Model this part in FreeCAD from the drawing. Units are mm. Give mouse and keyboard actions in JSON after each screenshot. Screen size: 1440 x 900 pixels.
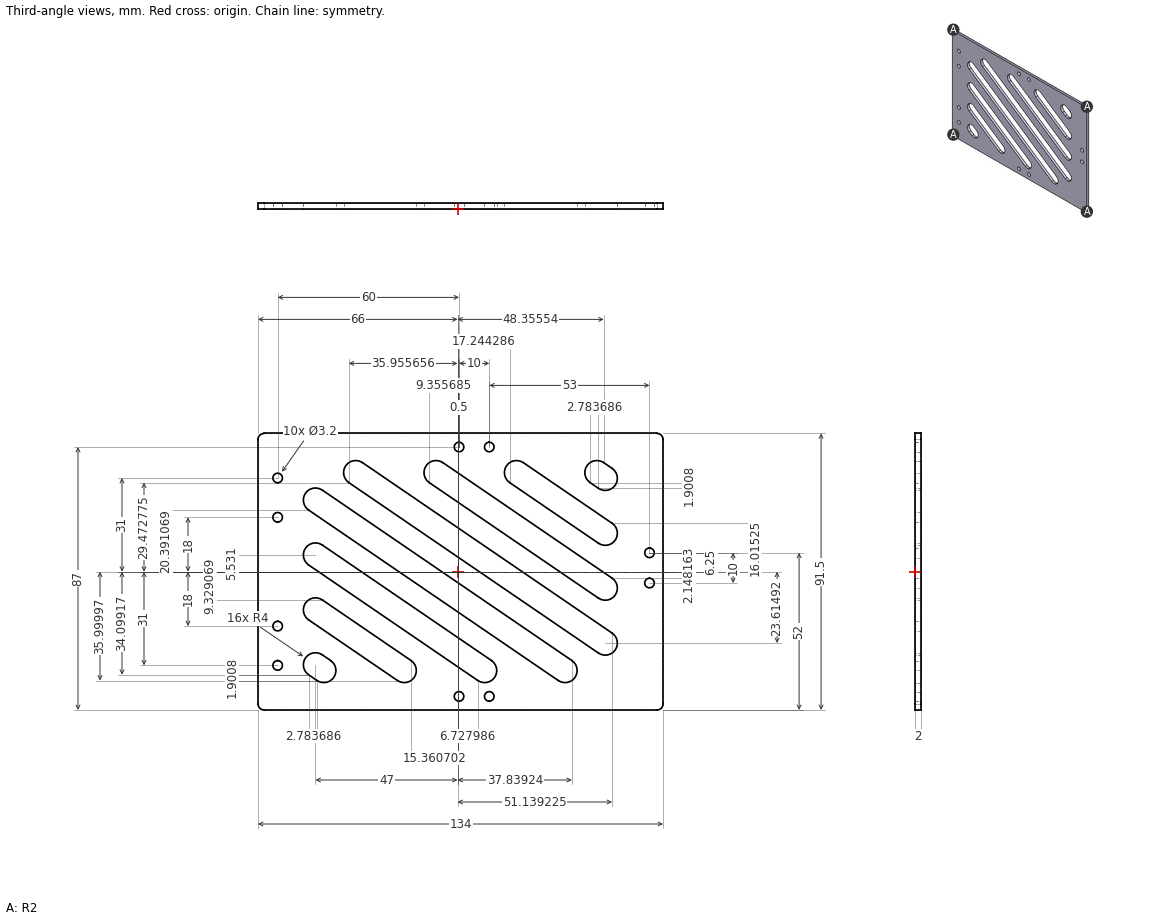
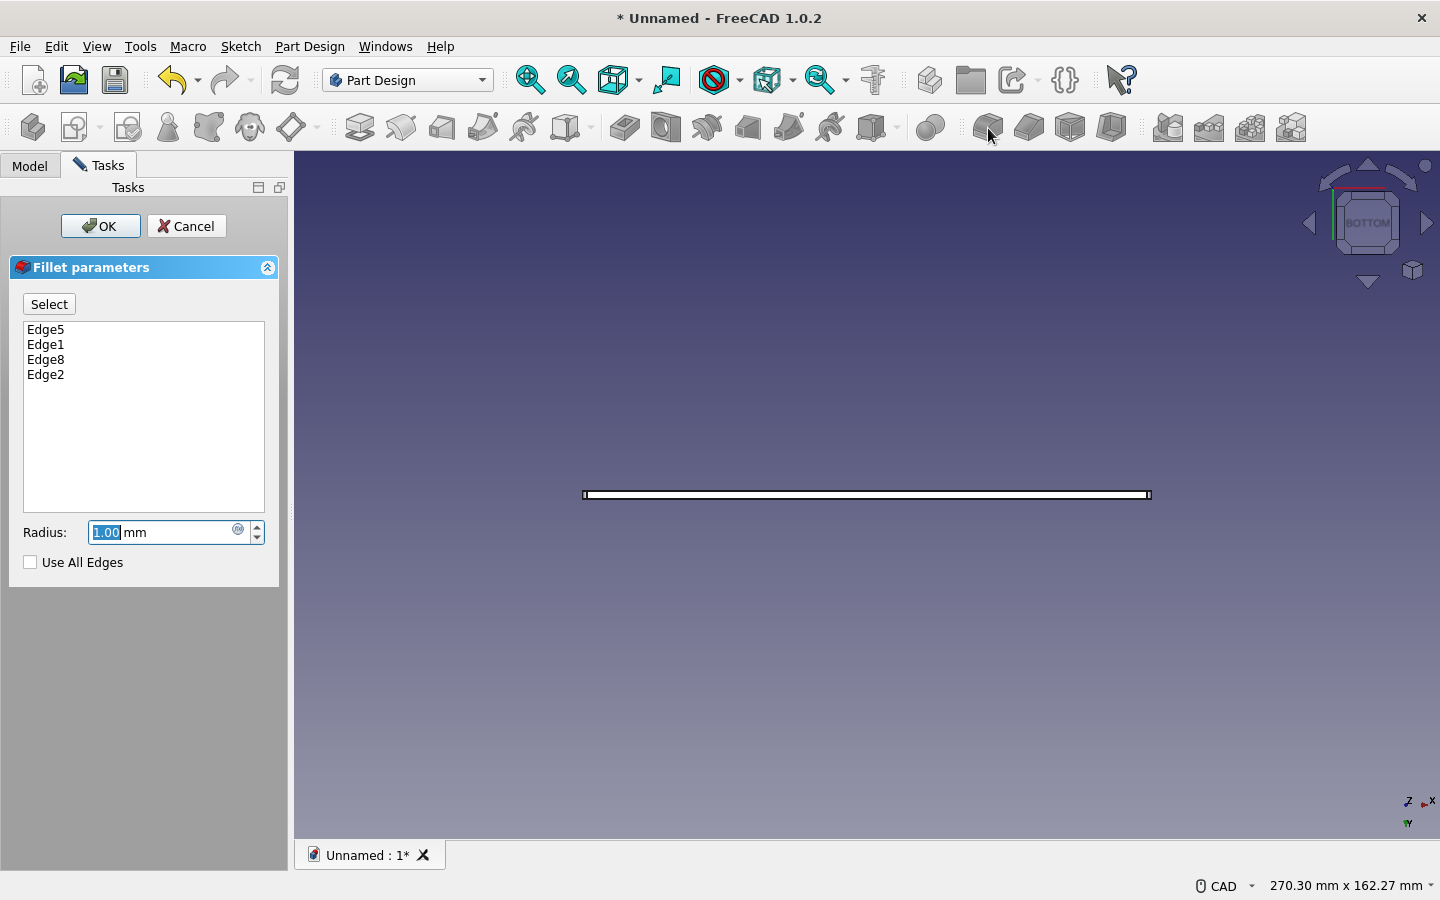
{"action": "type", "text": "2"}
{"action": "key", "text": "Tab"}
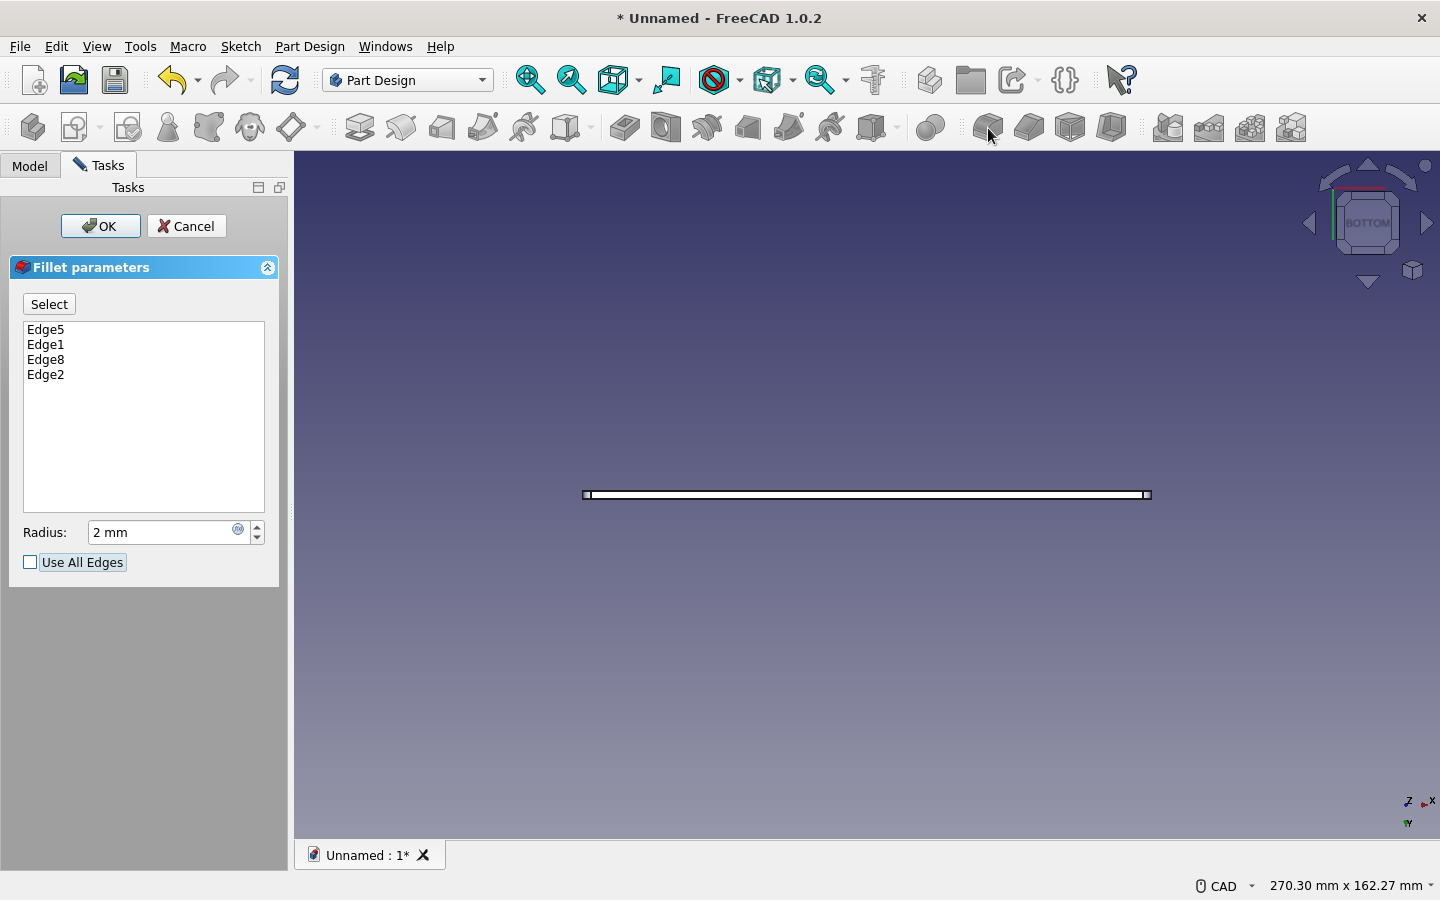
{"action": "left_click", "coordinate": [101, 226]}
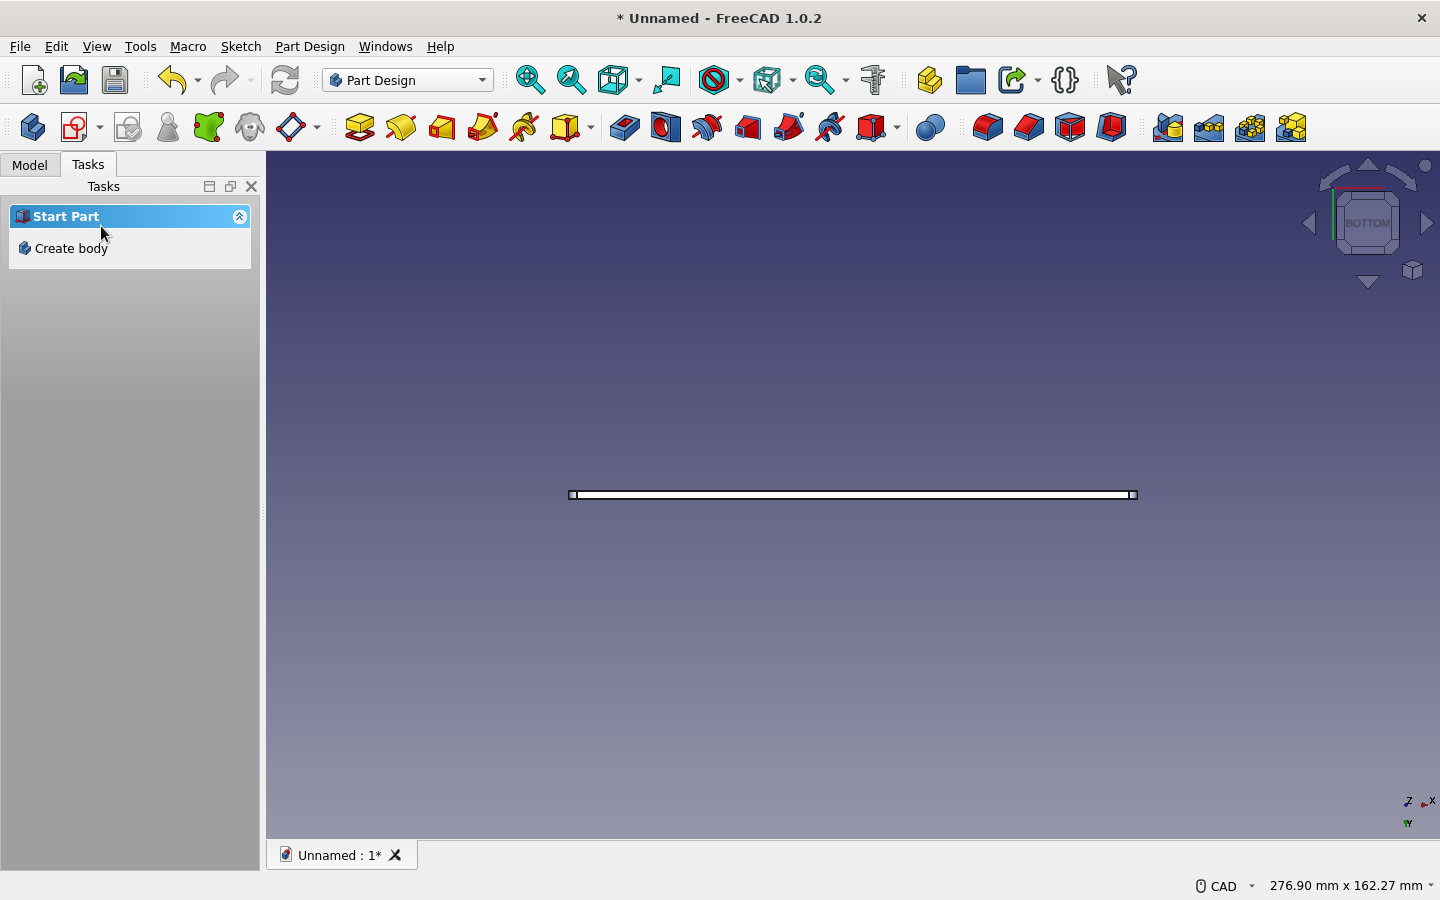
{"action": "key", "text": "0"}